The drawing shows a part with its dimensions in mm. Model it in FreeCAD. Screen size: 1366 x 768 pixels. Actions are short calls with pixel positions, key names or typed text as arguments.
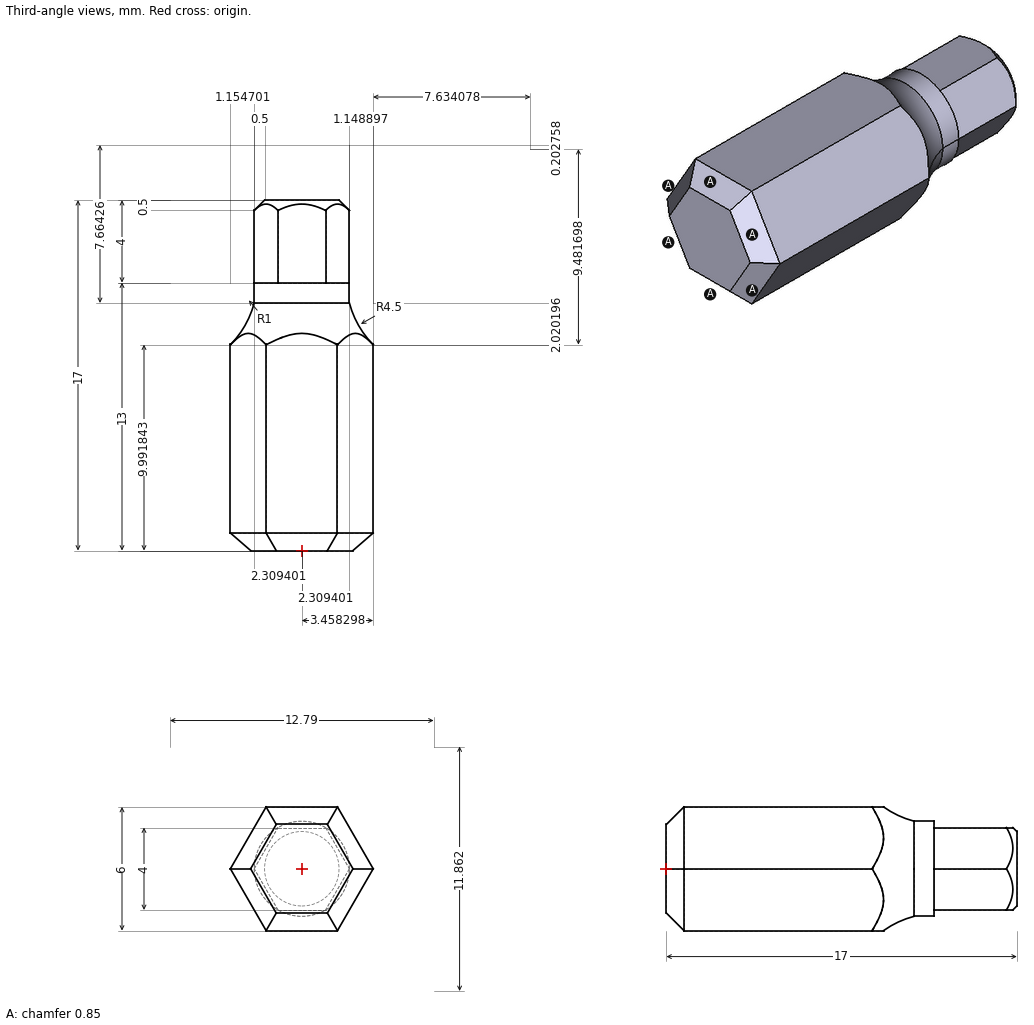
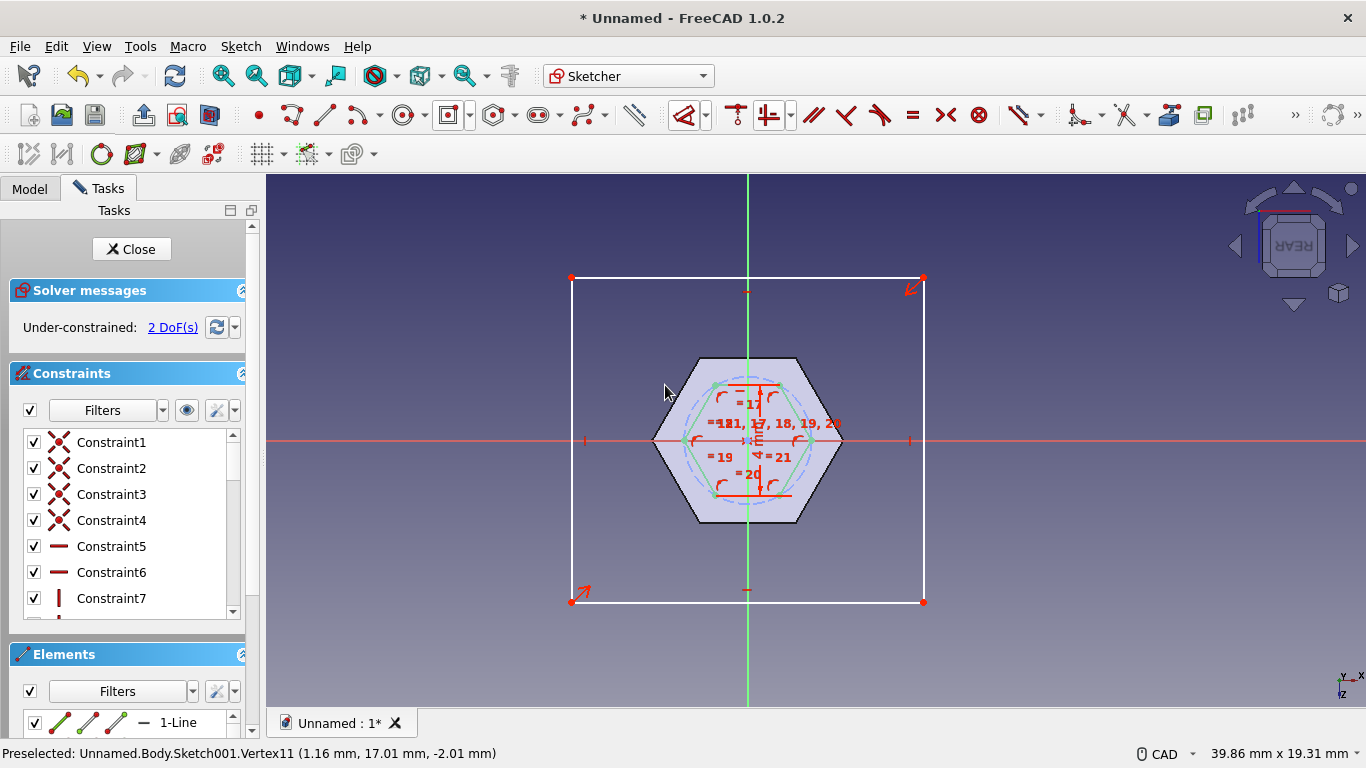
click(677, 603)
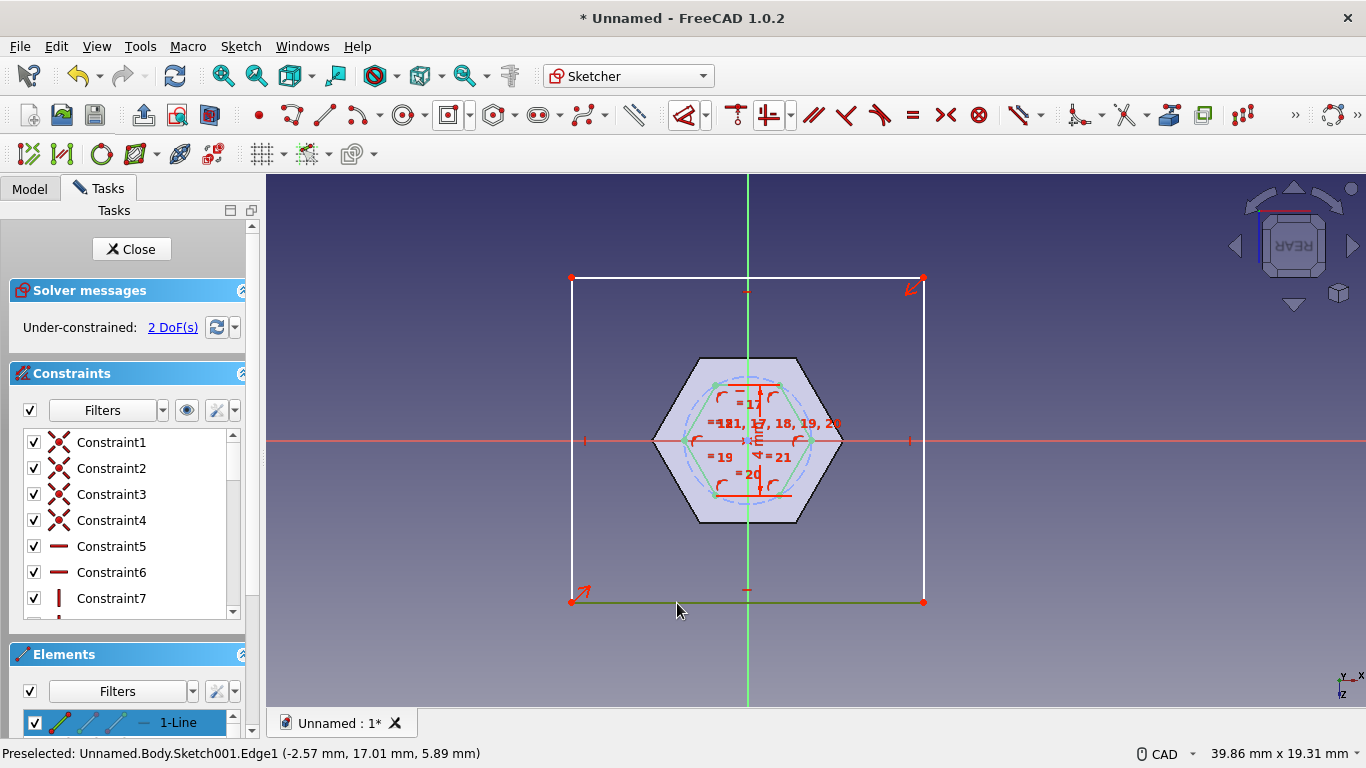
click(706, 116)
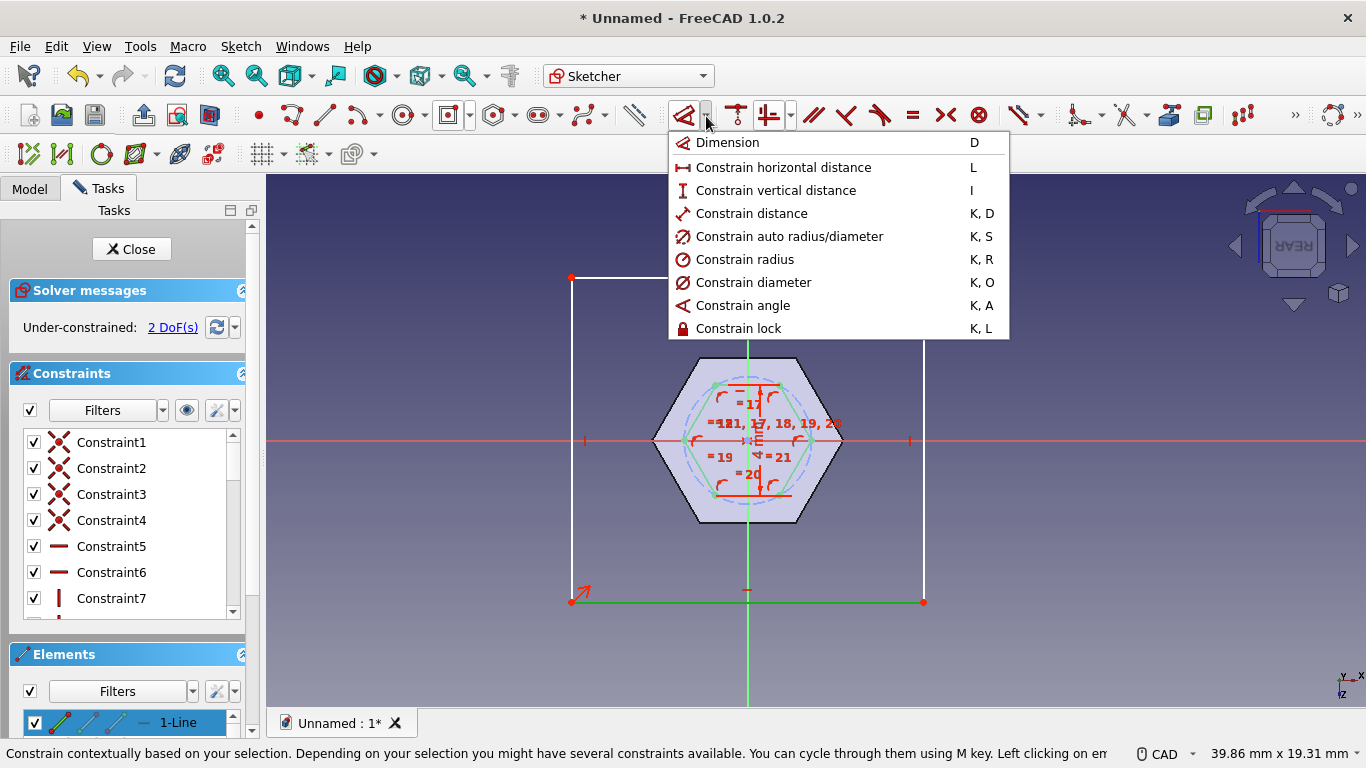
click(839, 168)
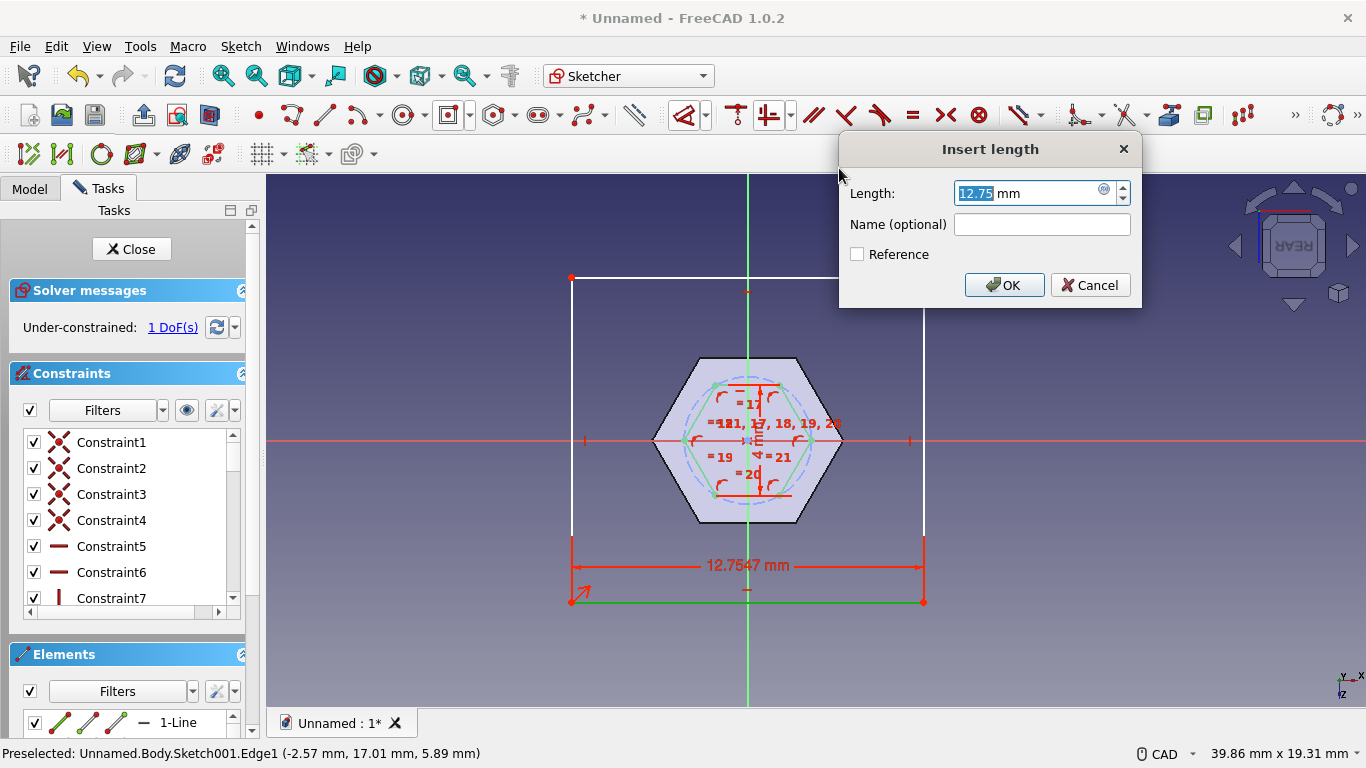
text(12.79)
key(Return)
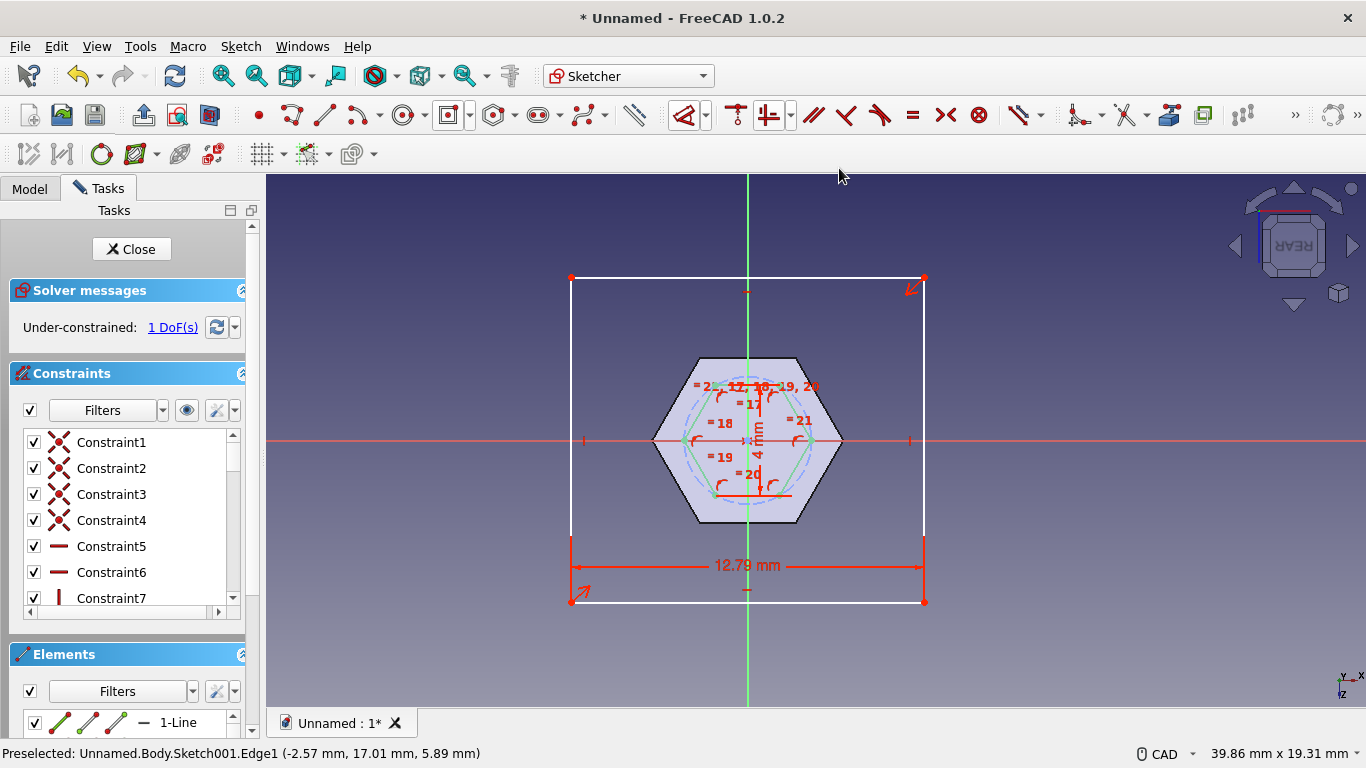
click(924, 505)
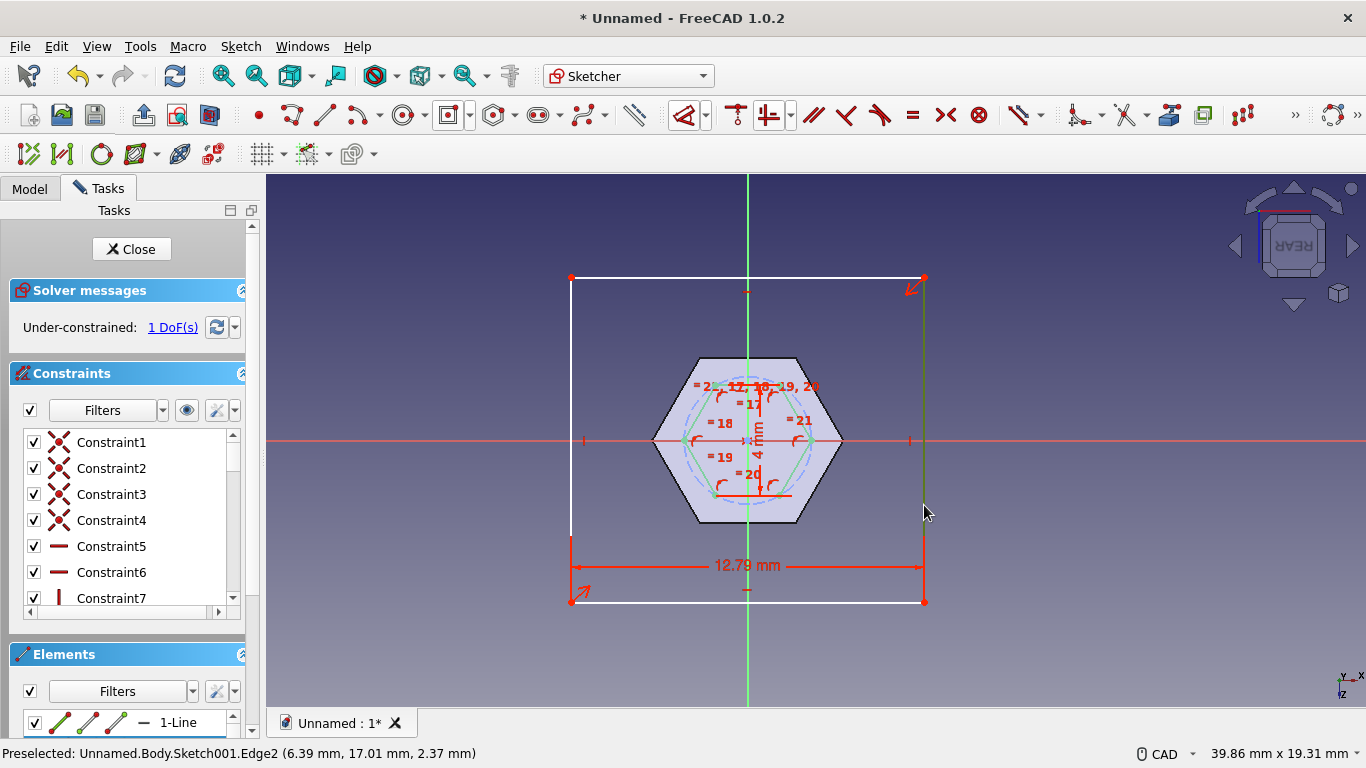
key(i)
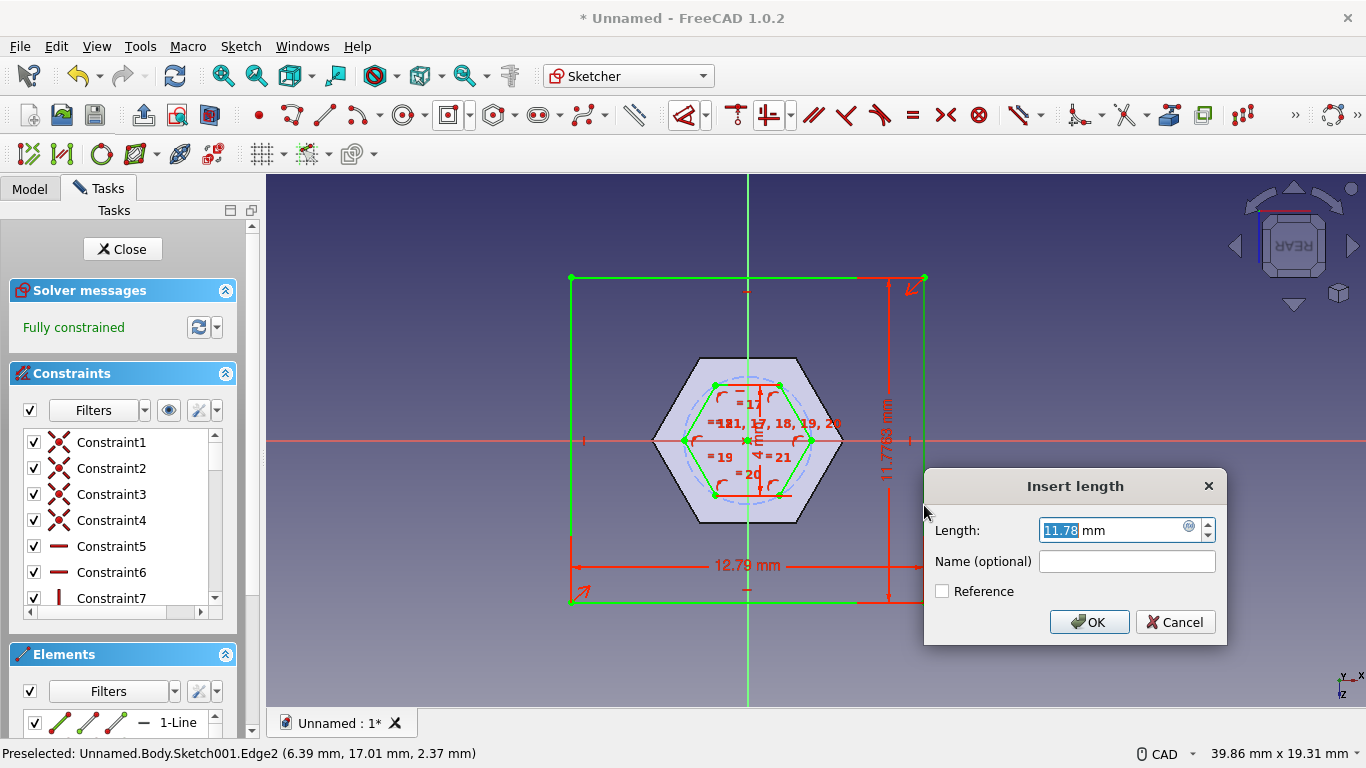
text(11.862)
key(Return)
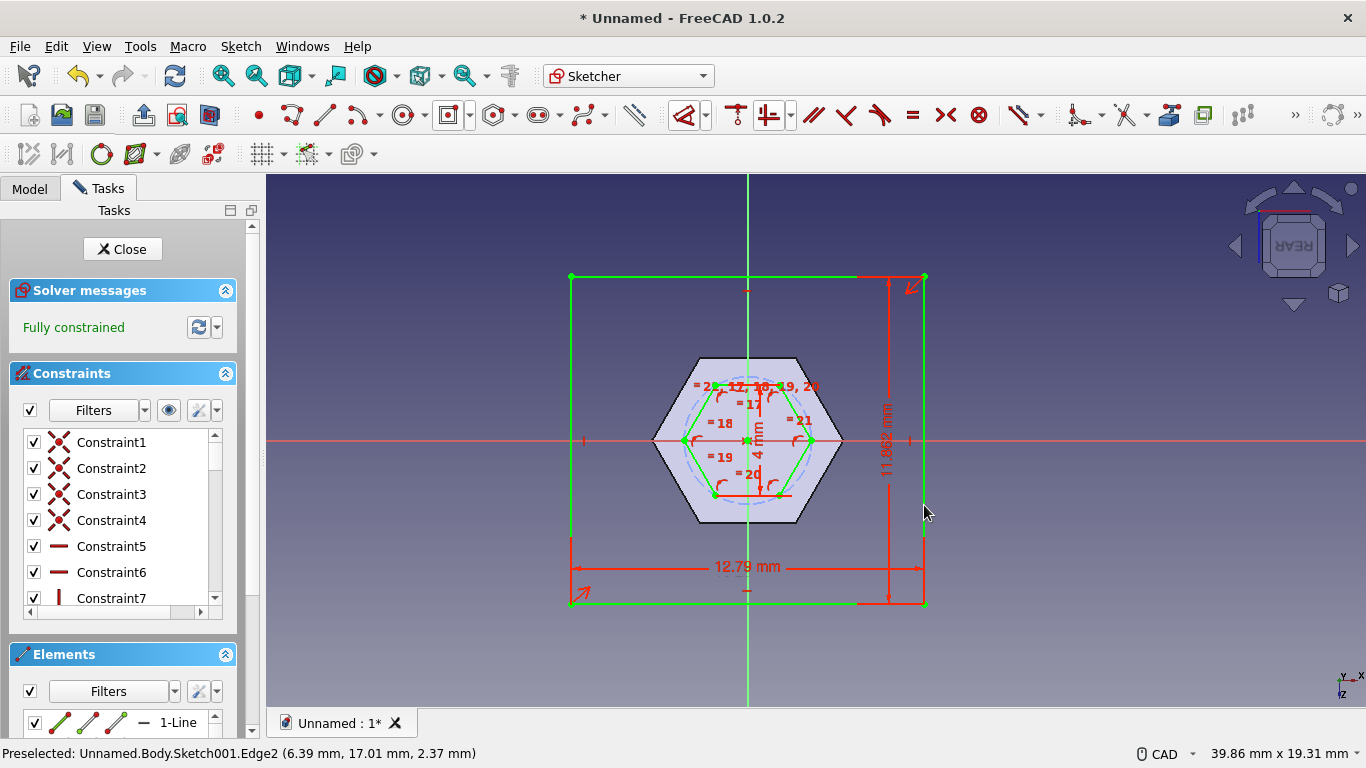
click(123, 249)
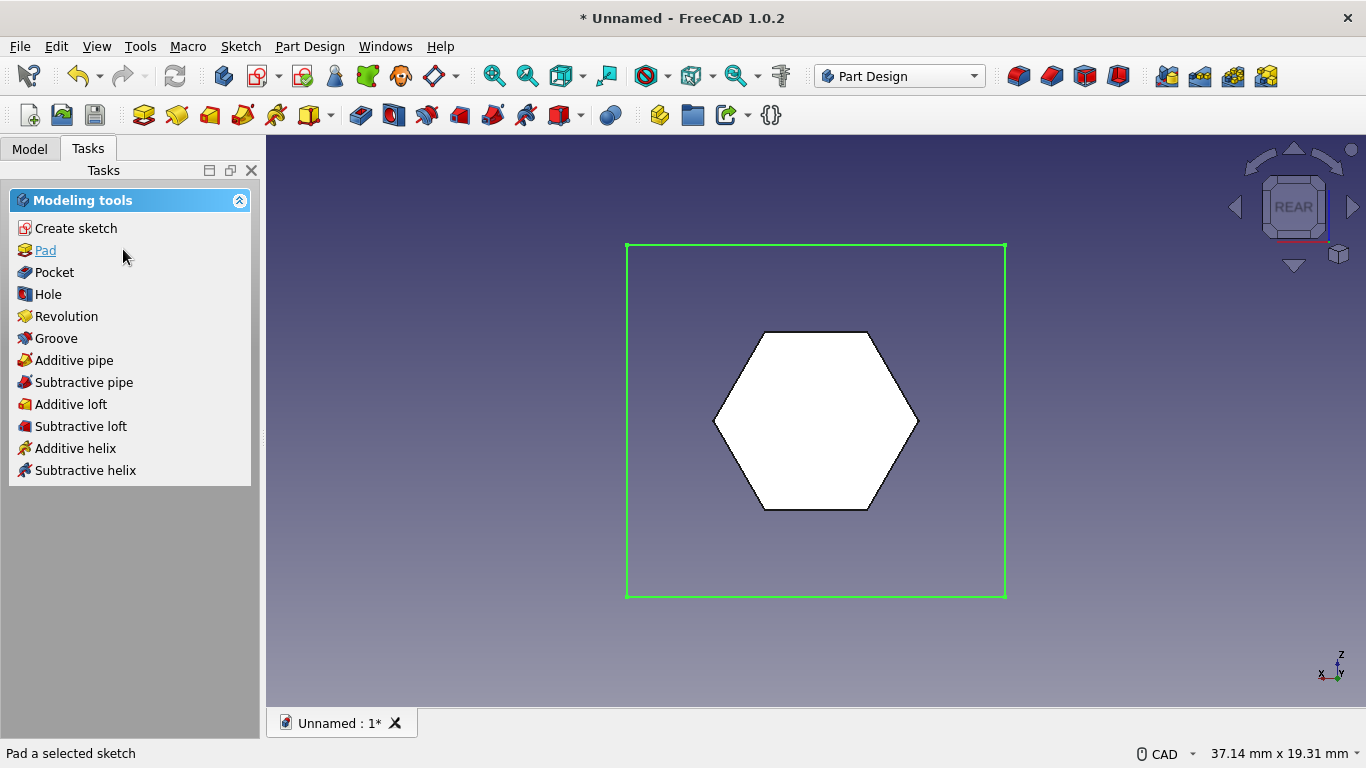
click(361, 116)